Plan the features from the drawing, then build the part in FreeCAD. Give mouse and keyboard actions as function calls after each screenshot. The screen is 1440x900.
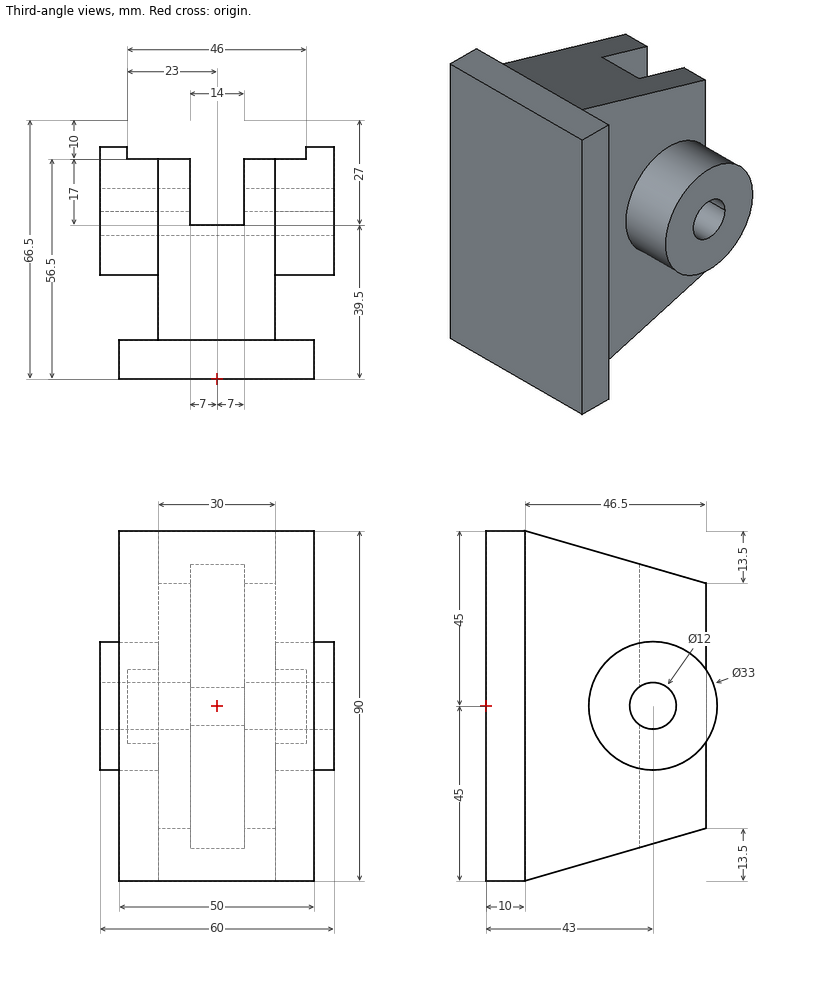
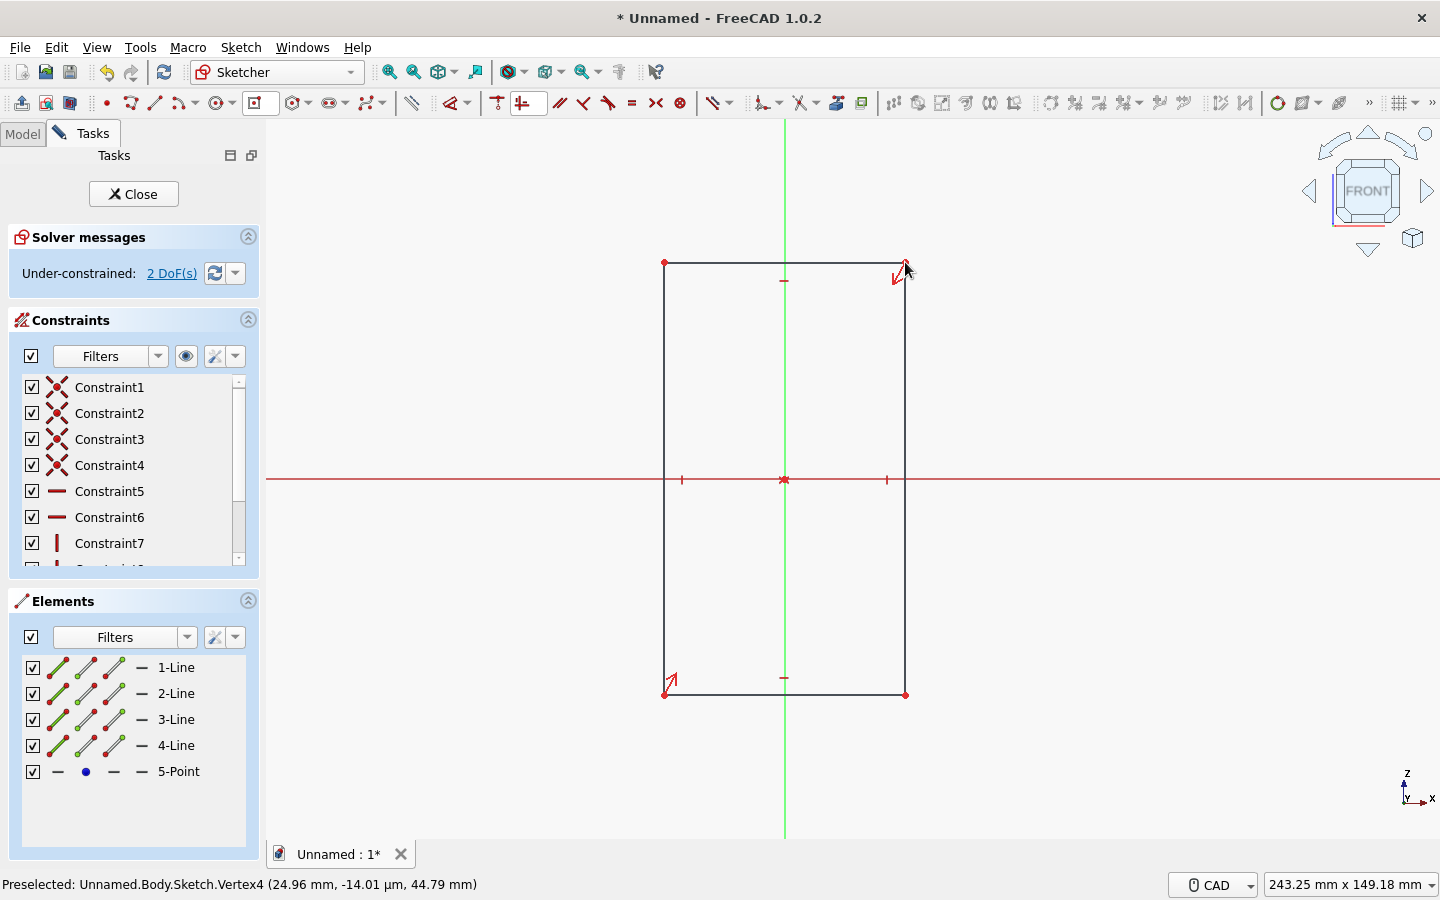
click(736, 695)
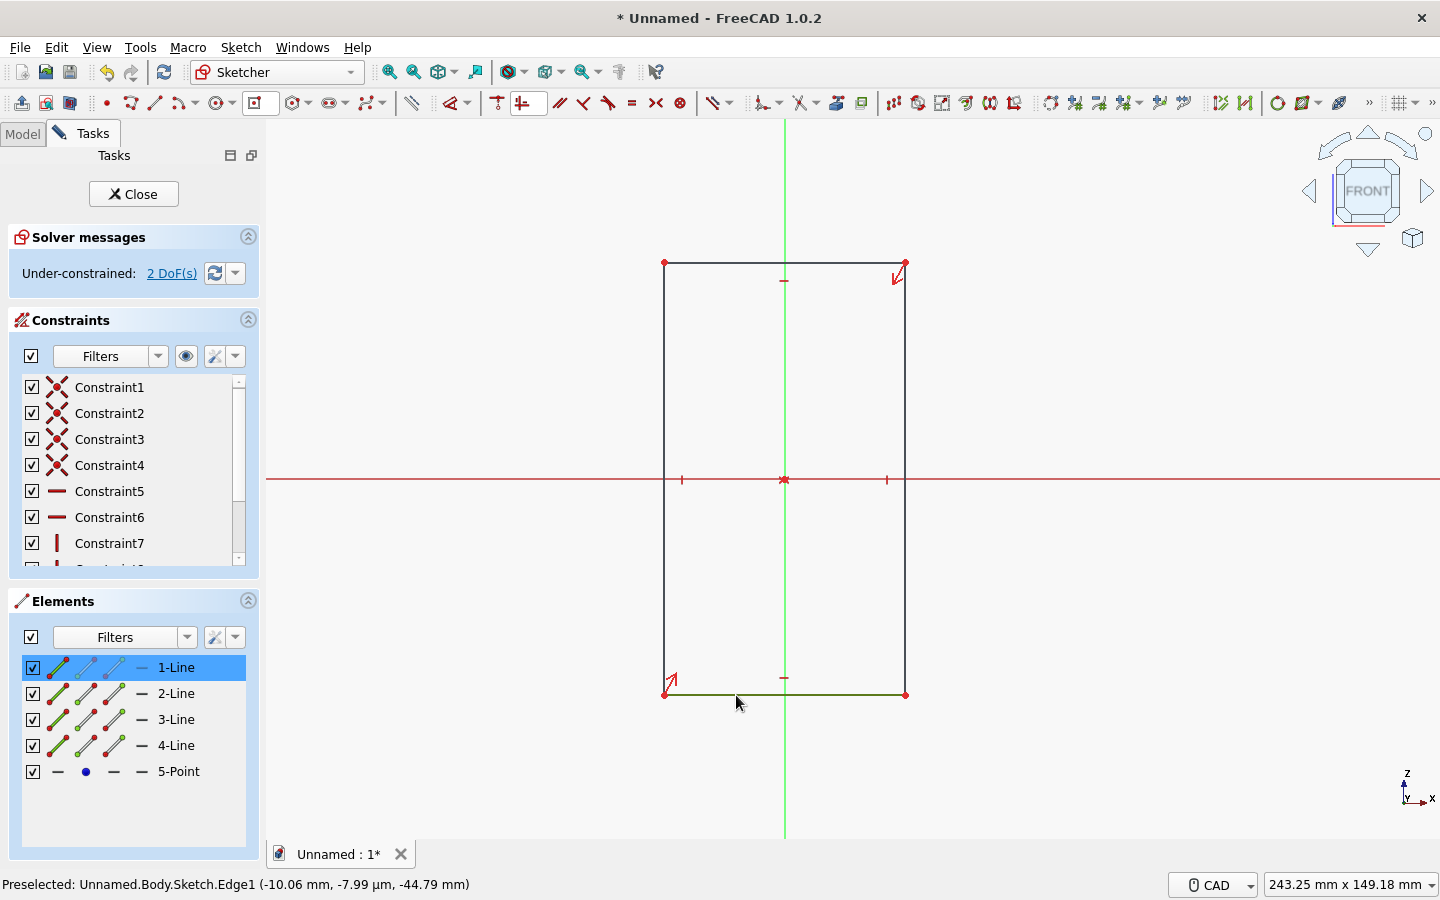
key(l)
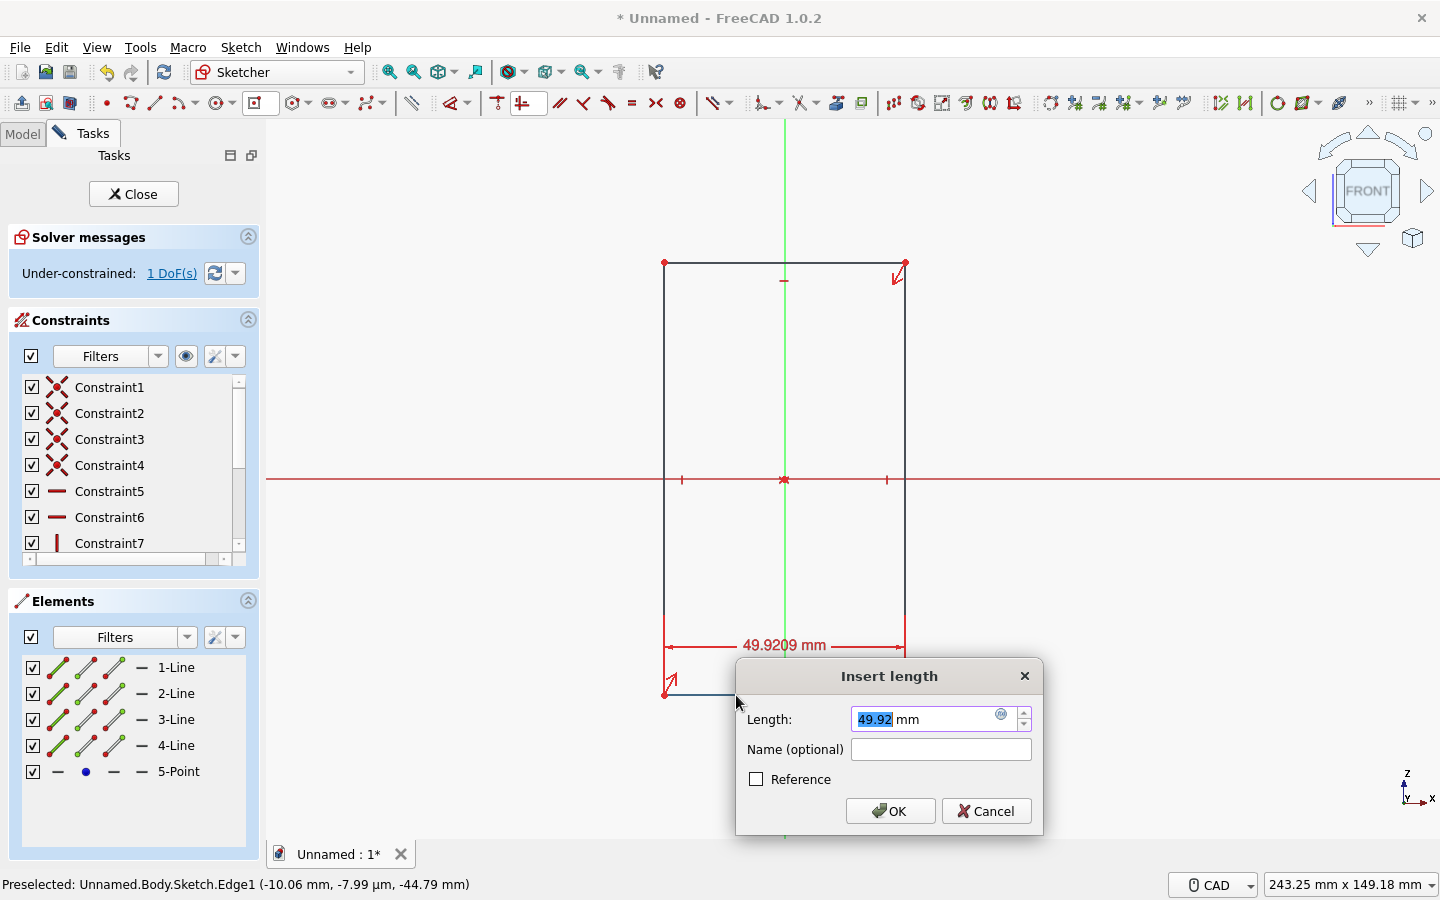
text(50)
key(Return)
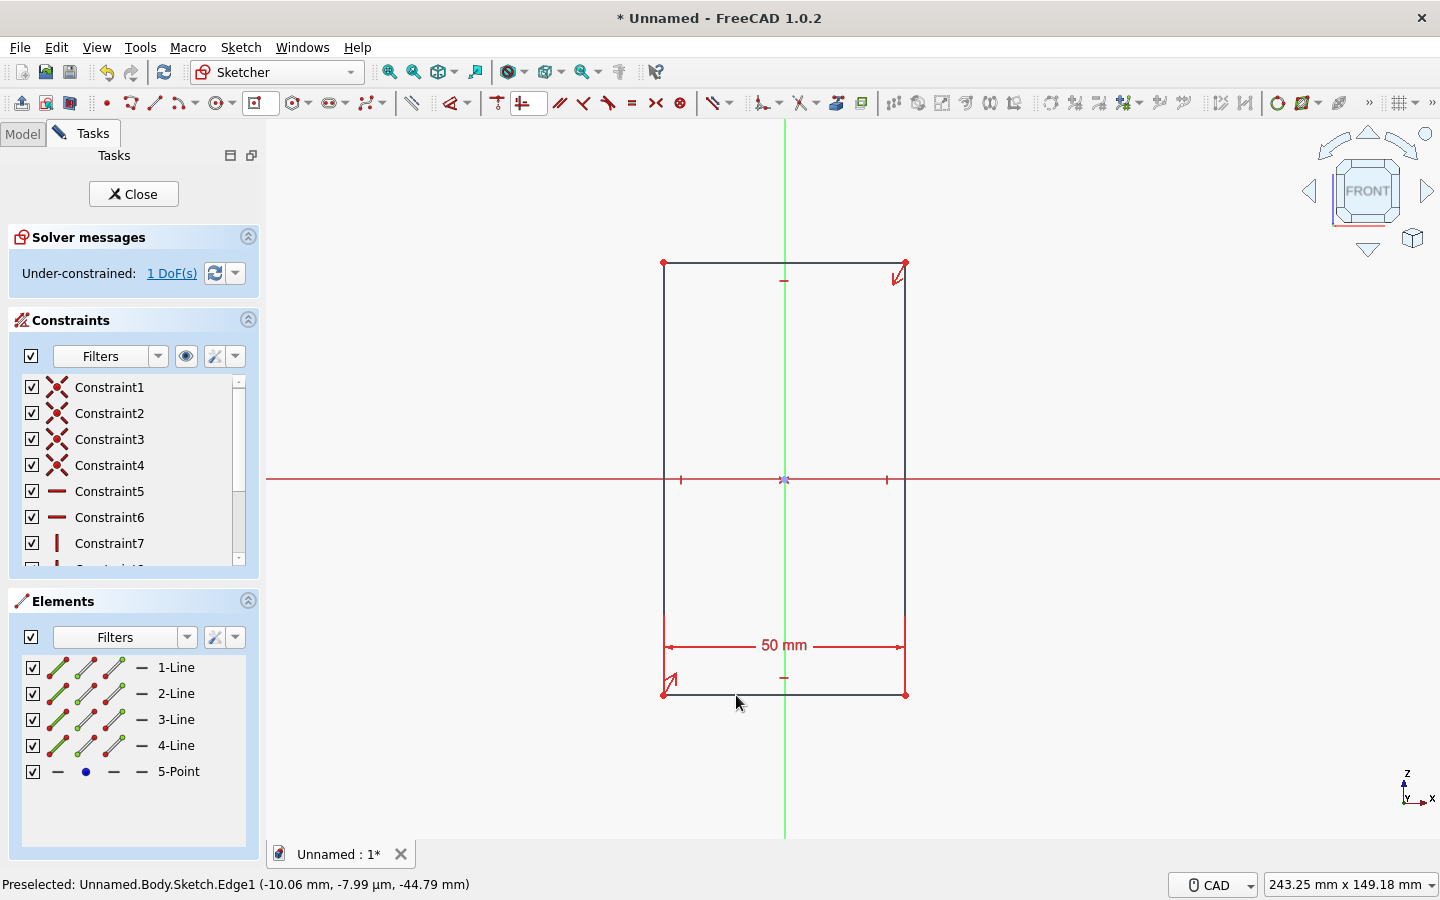
click(905, 566)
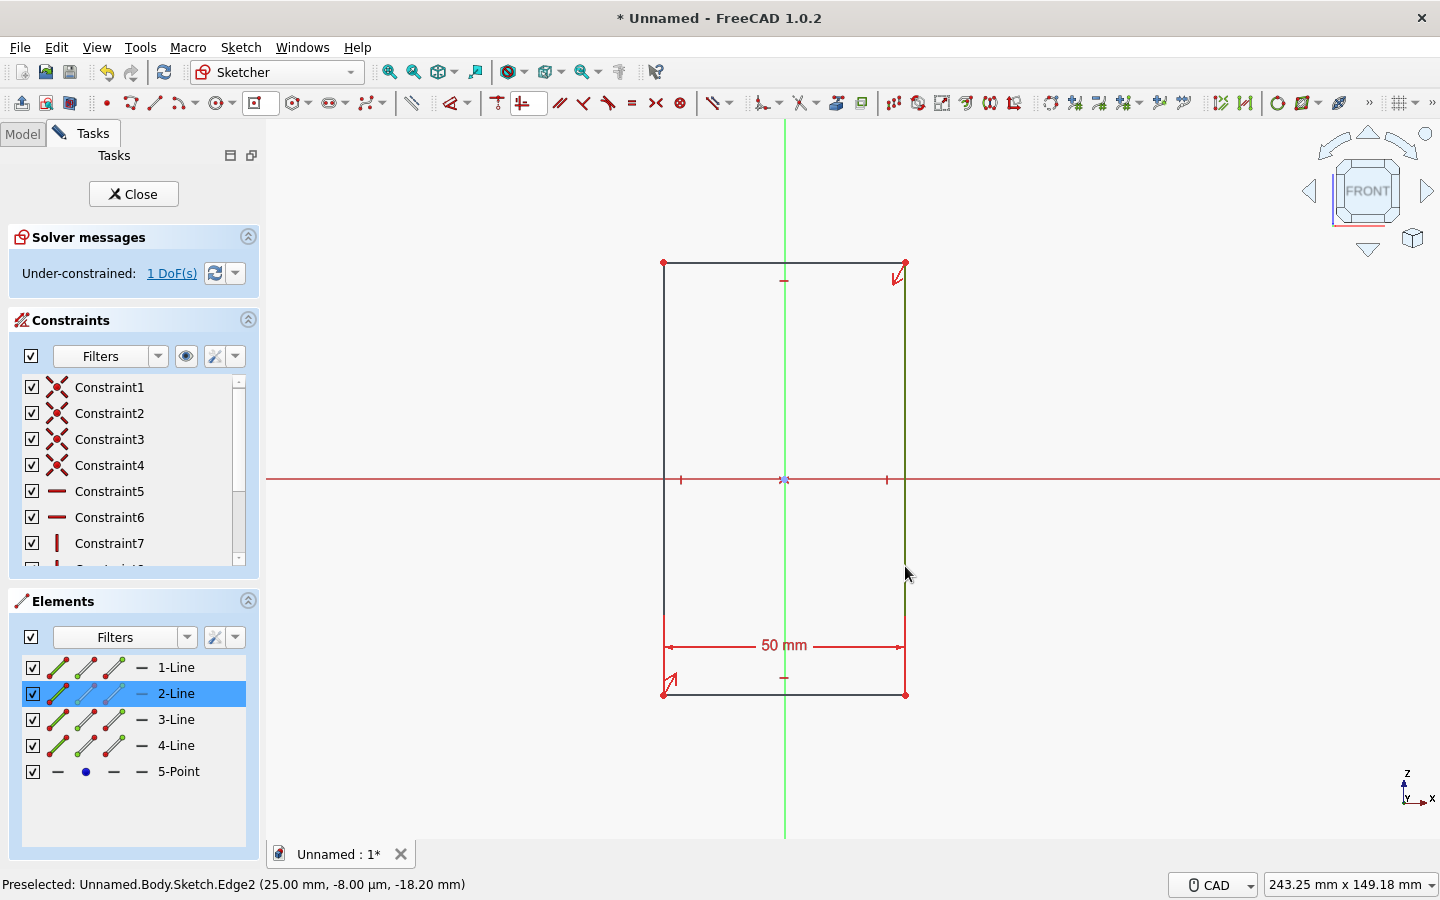
click(470, 104)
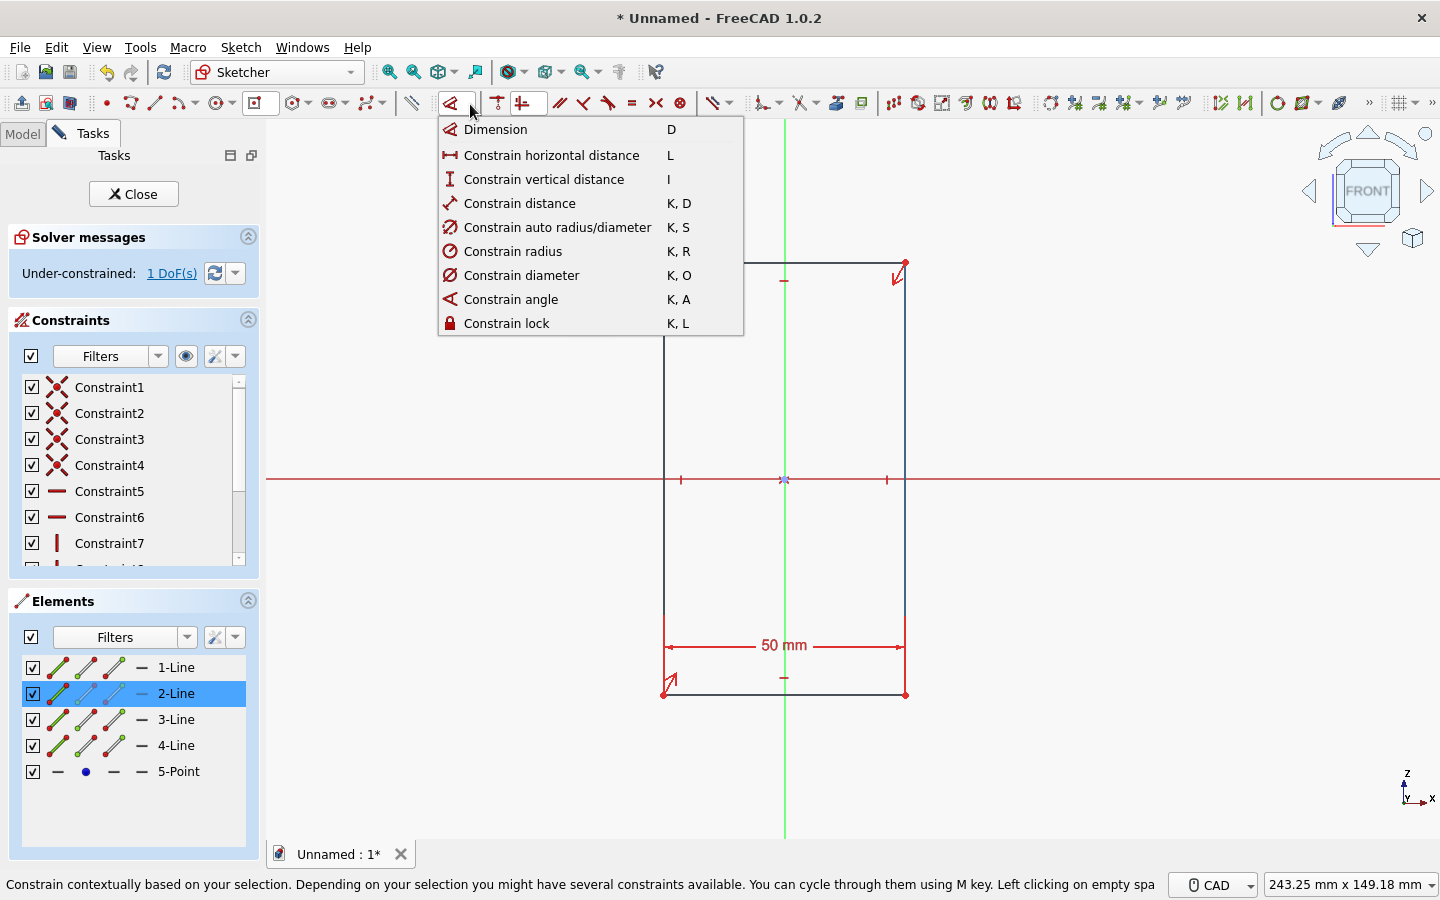
click(591, 179)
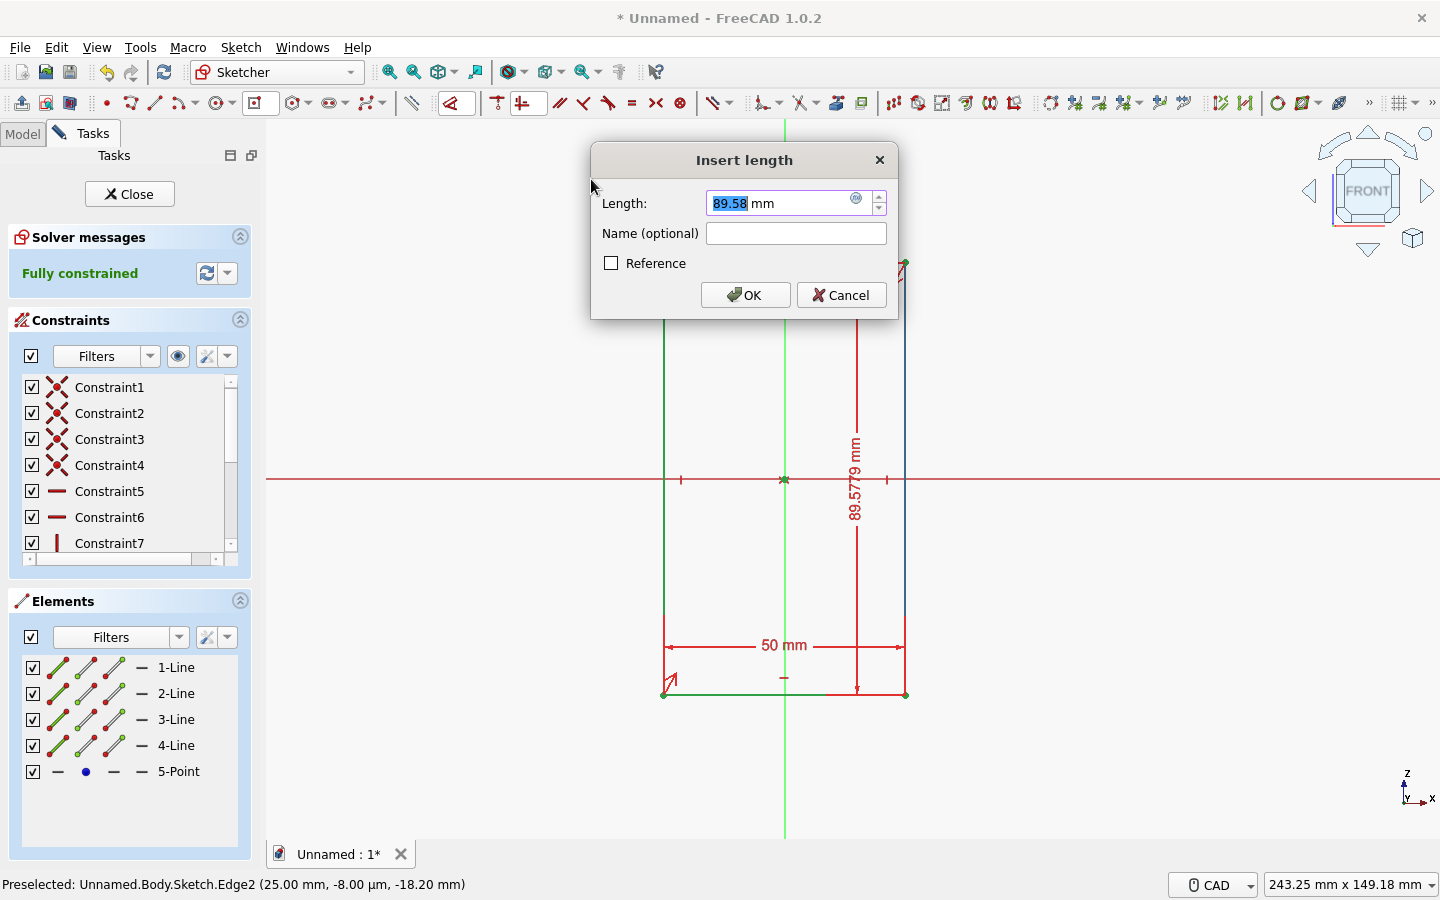
text(90)
key(Return)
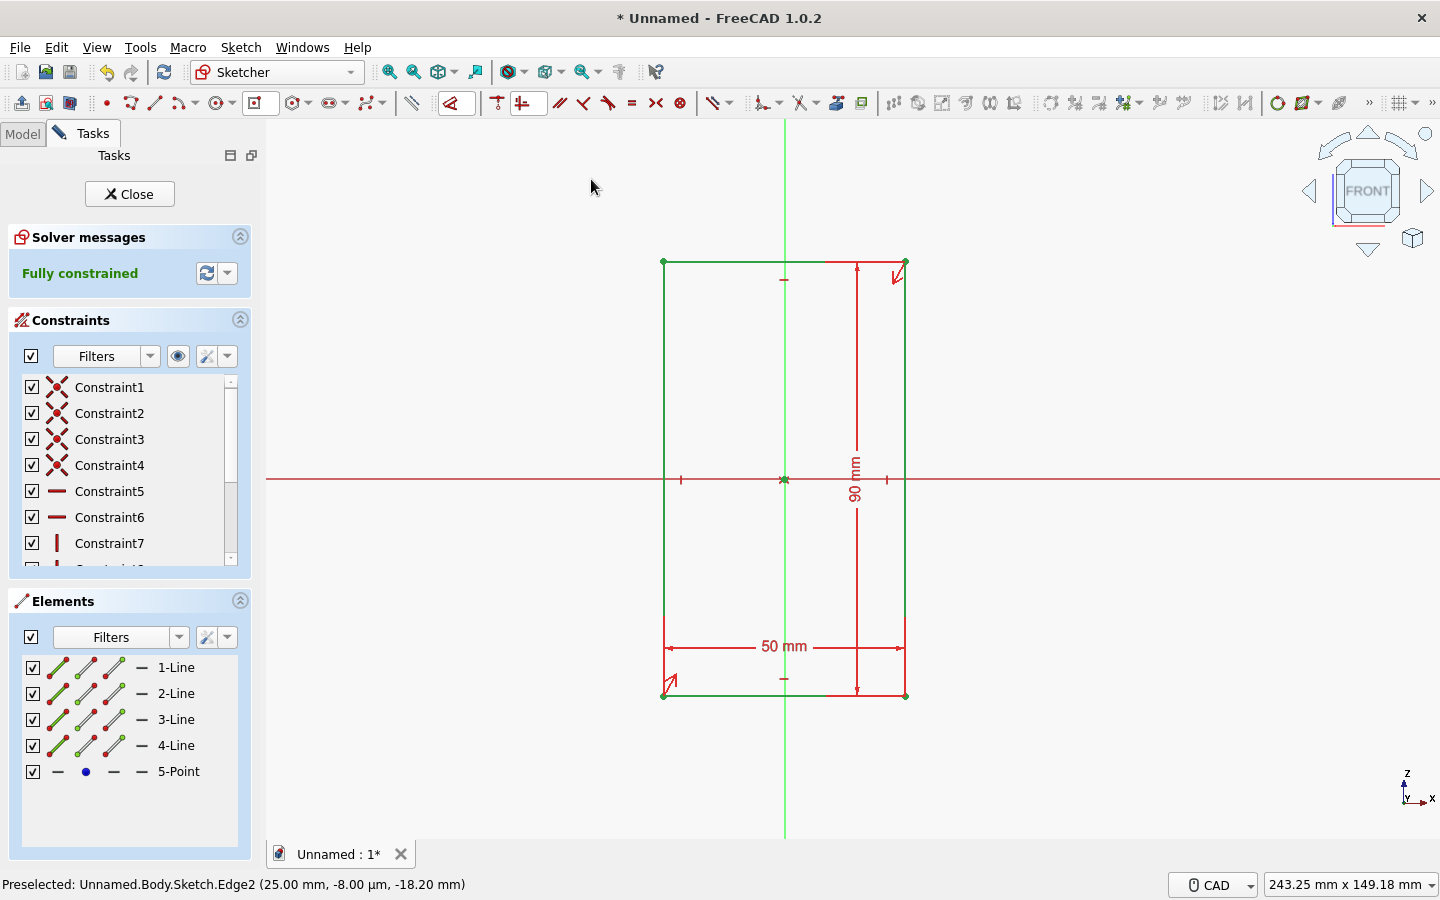
click(130, 194)